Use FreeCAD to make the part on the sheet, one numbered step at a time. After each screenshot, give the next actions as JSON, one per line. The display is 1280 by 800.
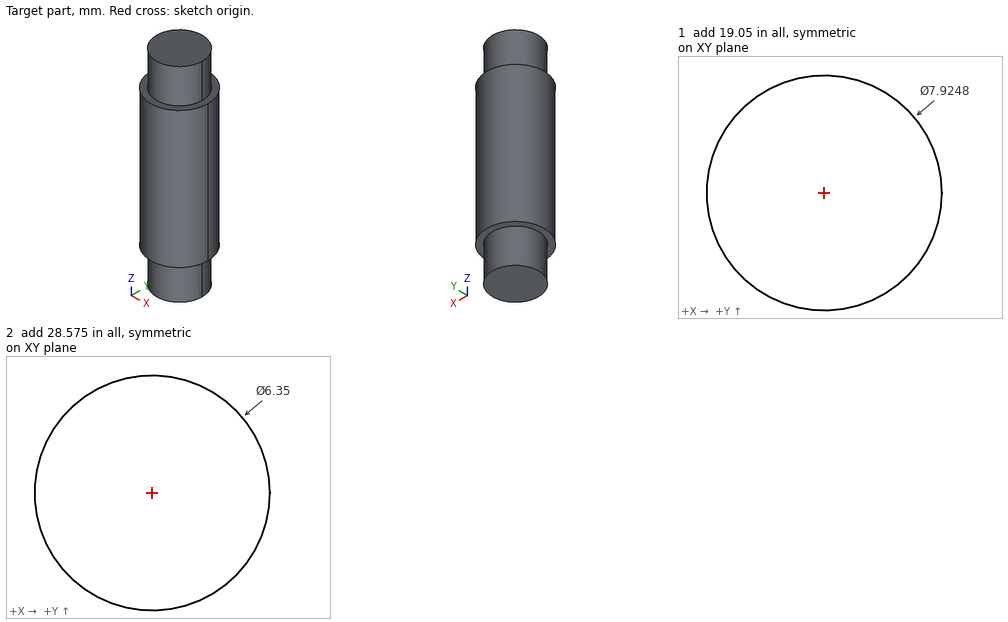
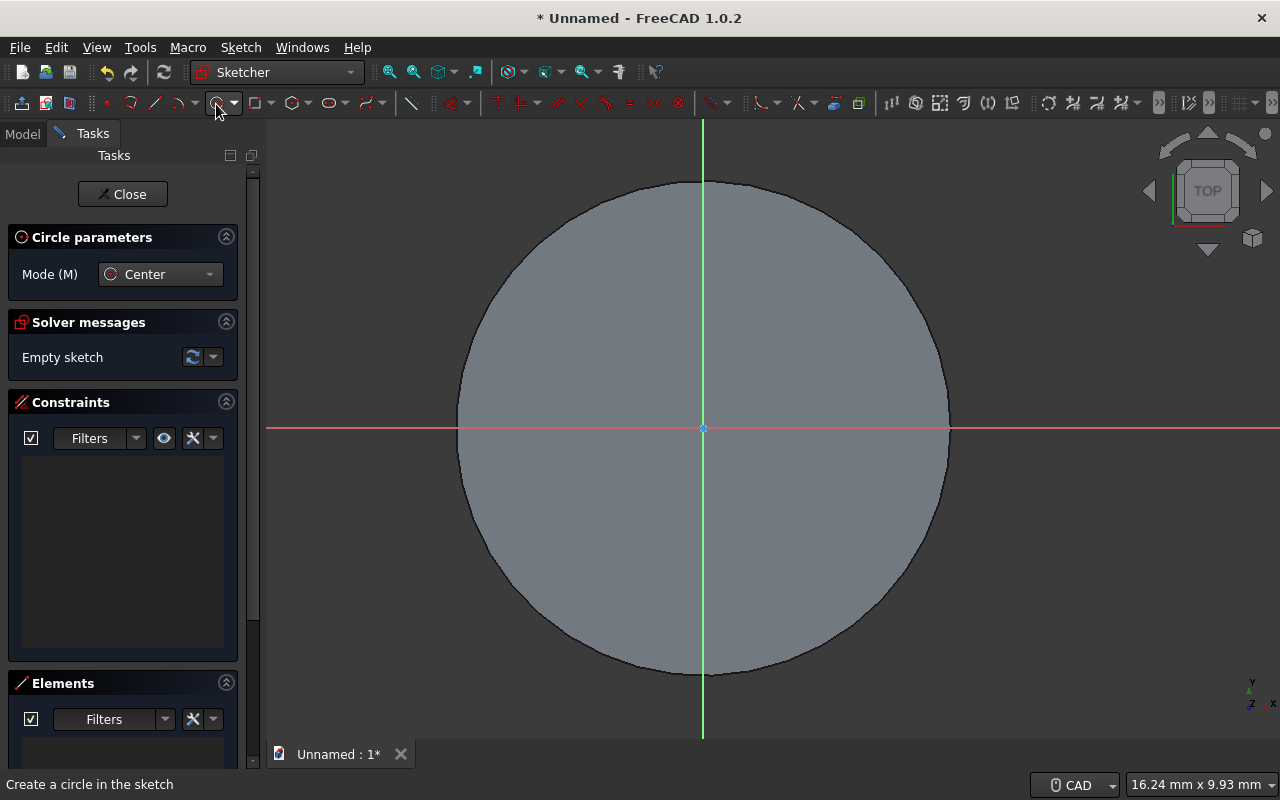
{"action": "left_click", "coordinate": [703, 428]}
{"action": "mouse_move", "coordinate": [844, 288]}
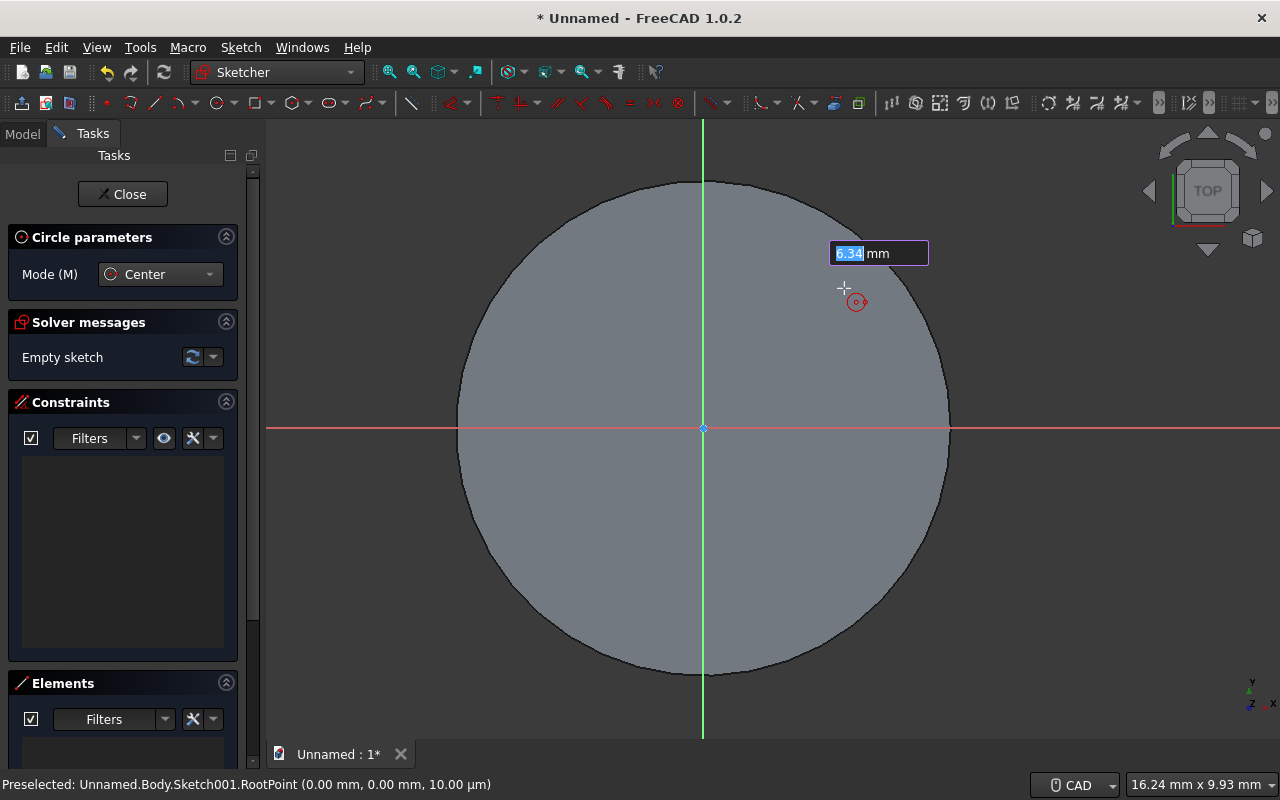
{"action": "type", "text": "6.35"}
{"action": "key", "text": "Return"}
{"action": "key", "text": "Escape"}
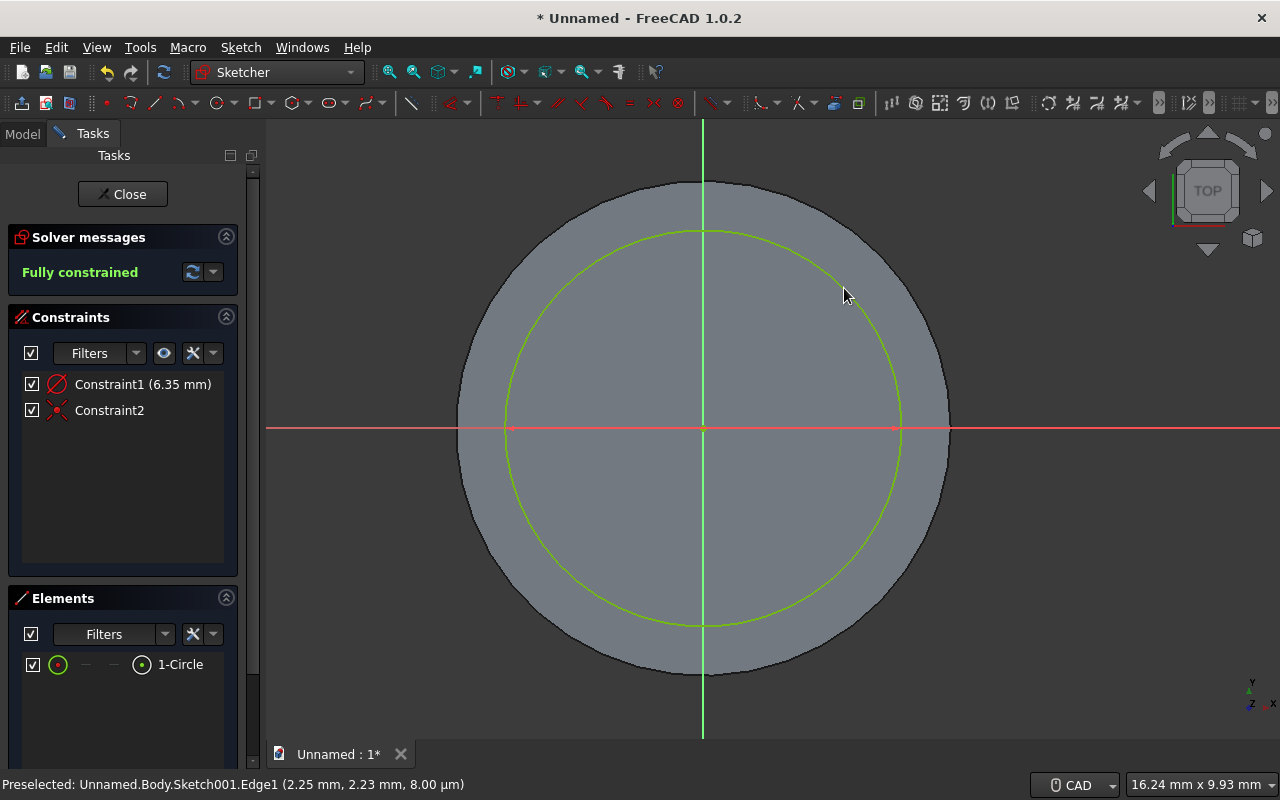
{"action": "left_click", "coordinate": [123, 194]}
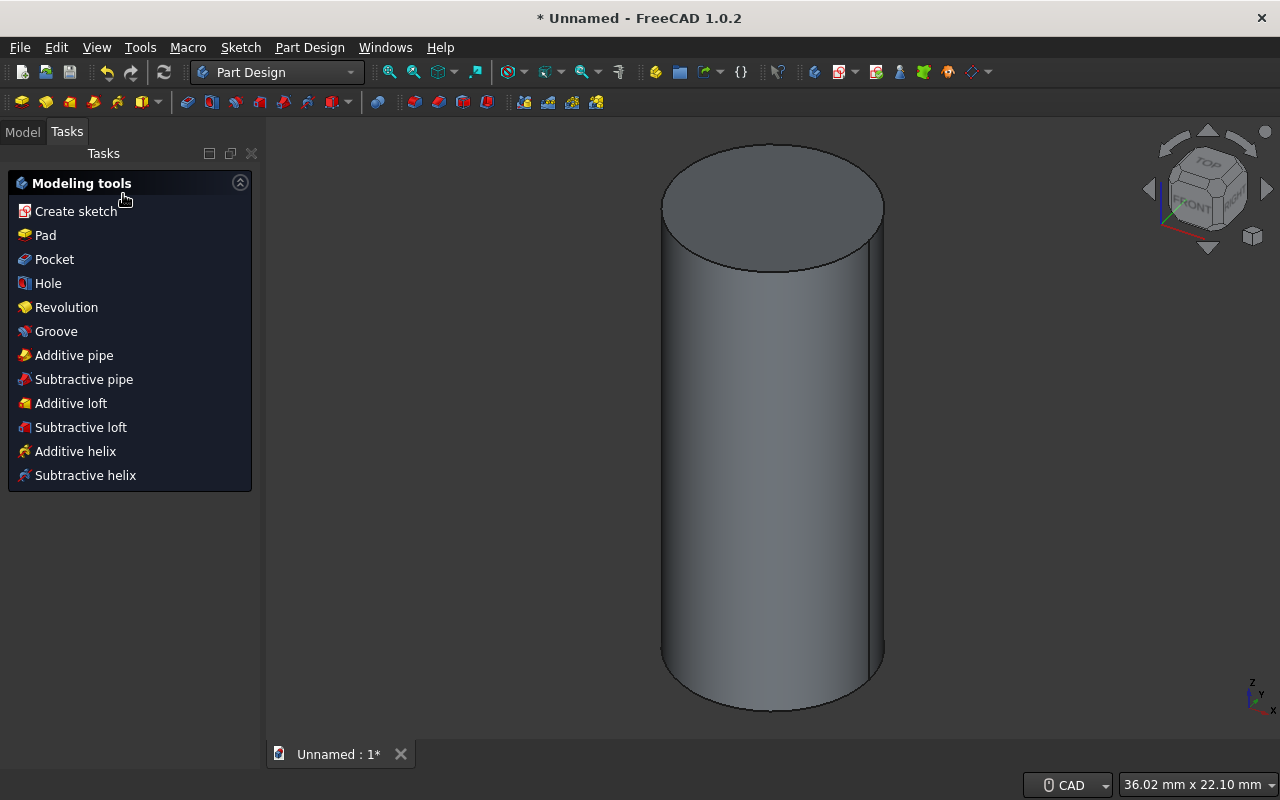
{"action": "left_click", "coordinate": [22, 102]}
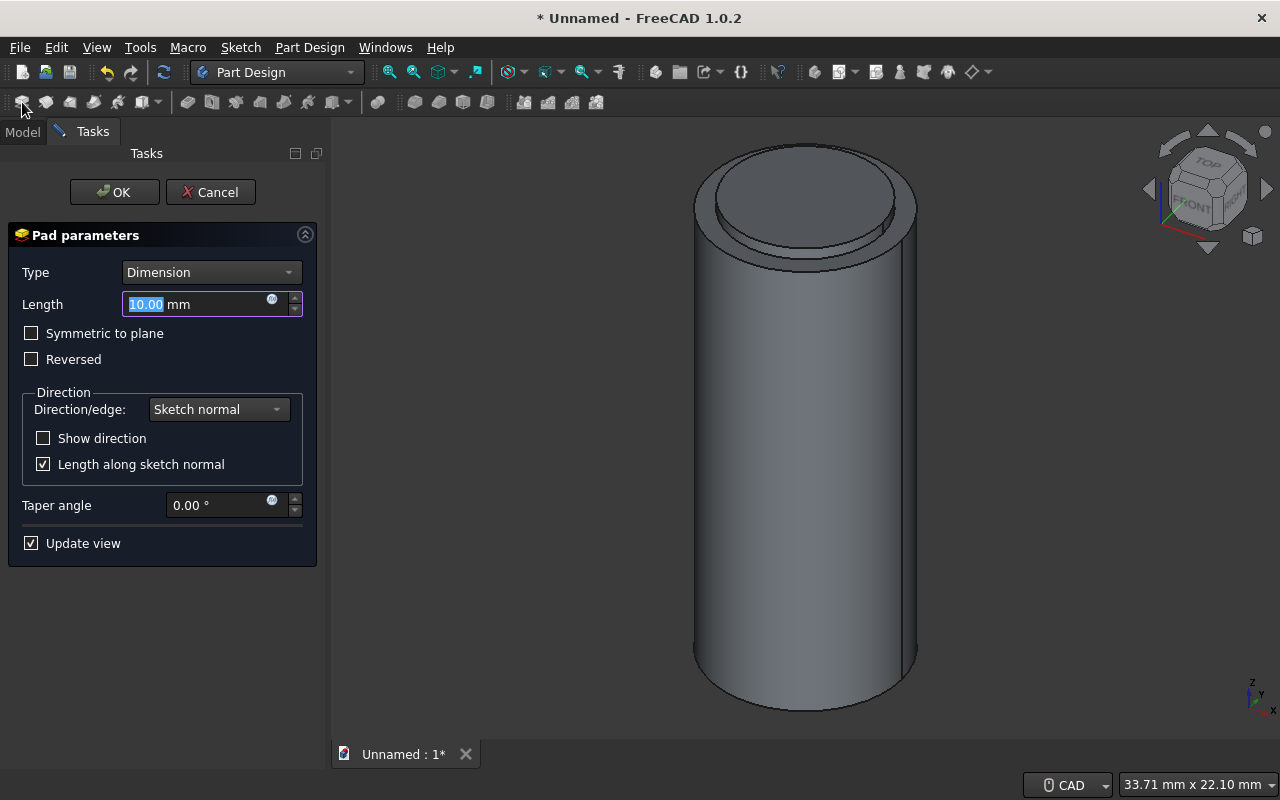
{"action": "type", "text": "28.575"}
{"action": "key", "text": "Tab"}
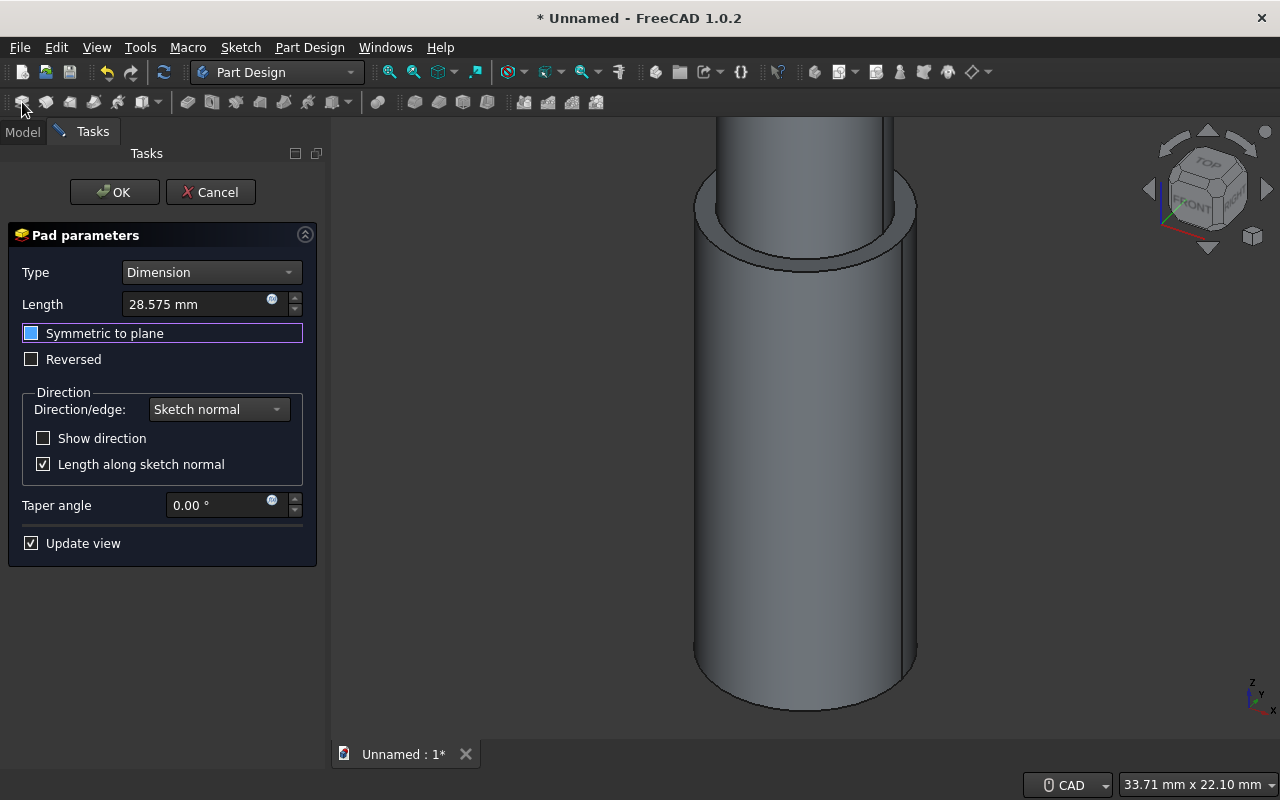
{"action": "left_click", "coordinate": [30, 333]}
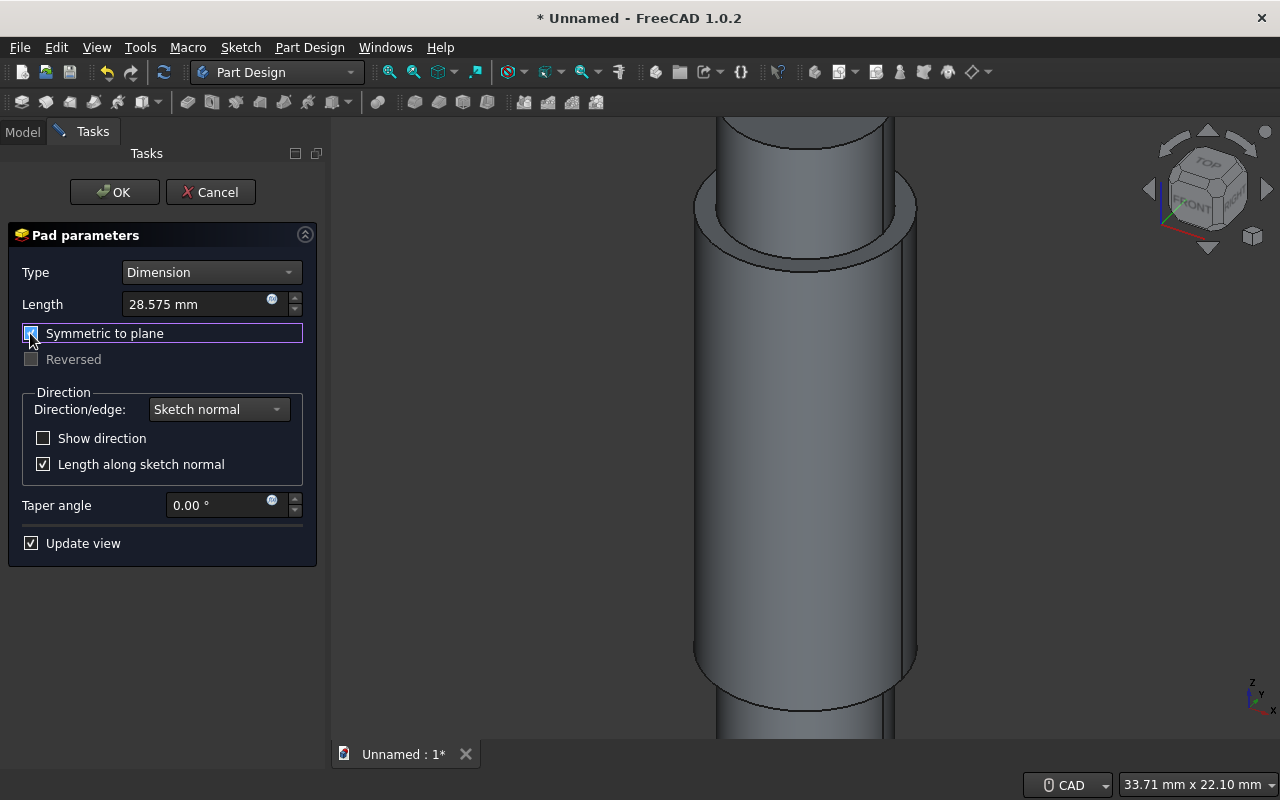
{"action": "left_click", "coordinate": [115, 192]}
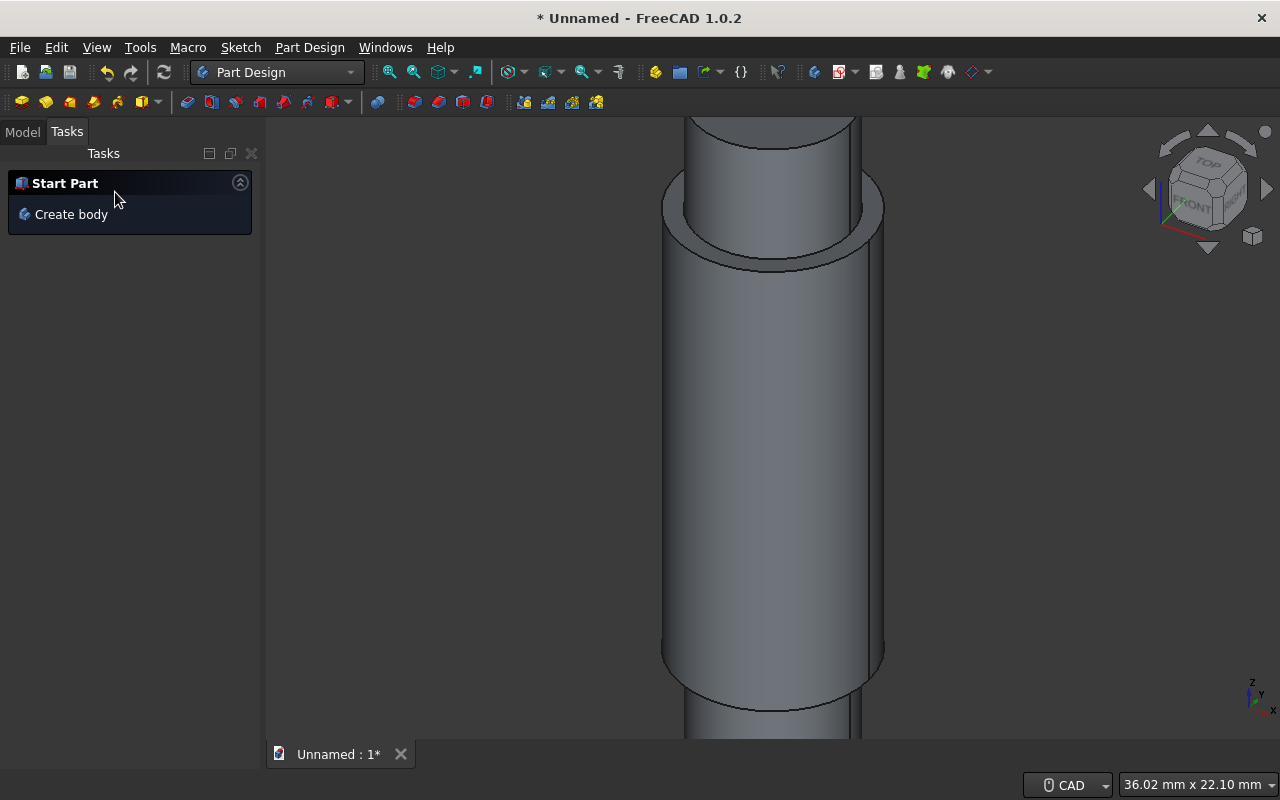
{"action": "key", "text": "0"}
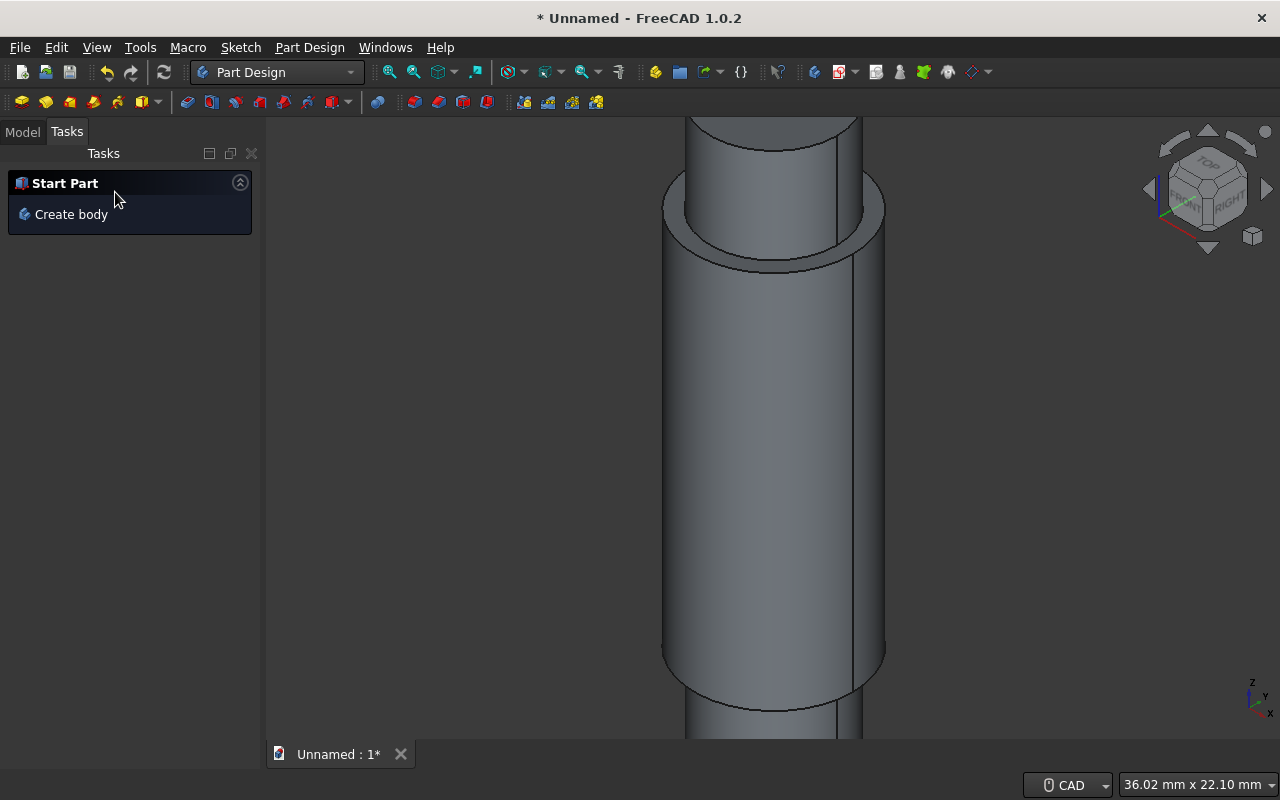
{"action": "left_click", "coordinate": [390, 72]}